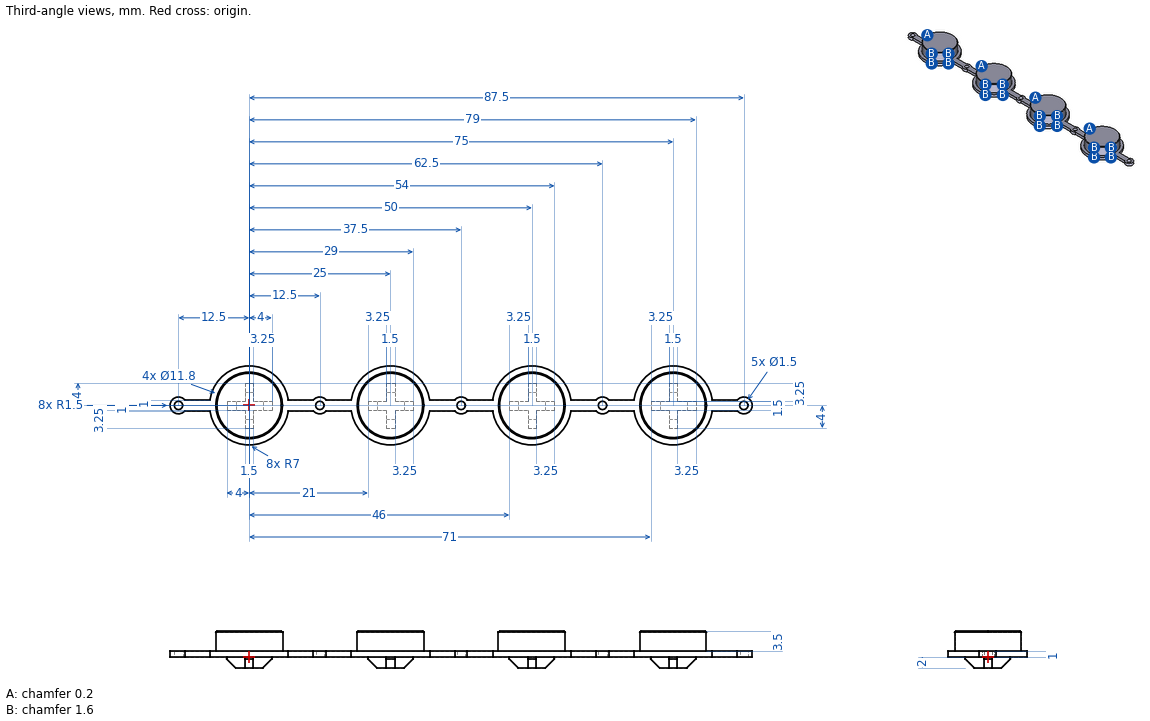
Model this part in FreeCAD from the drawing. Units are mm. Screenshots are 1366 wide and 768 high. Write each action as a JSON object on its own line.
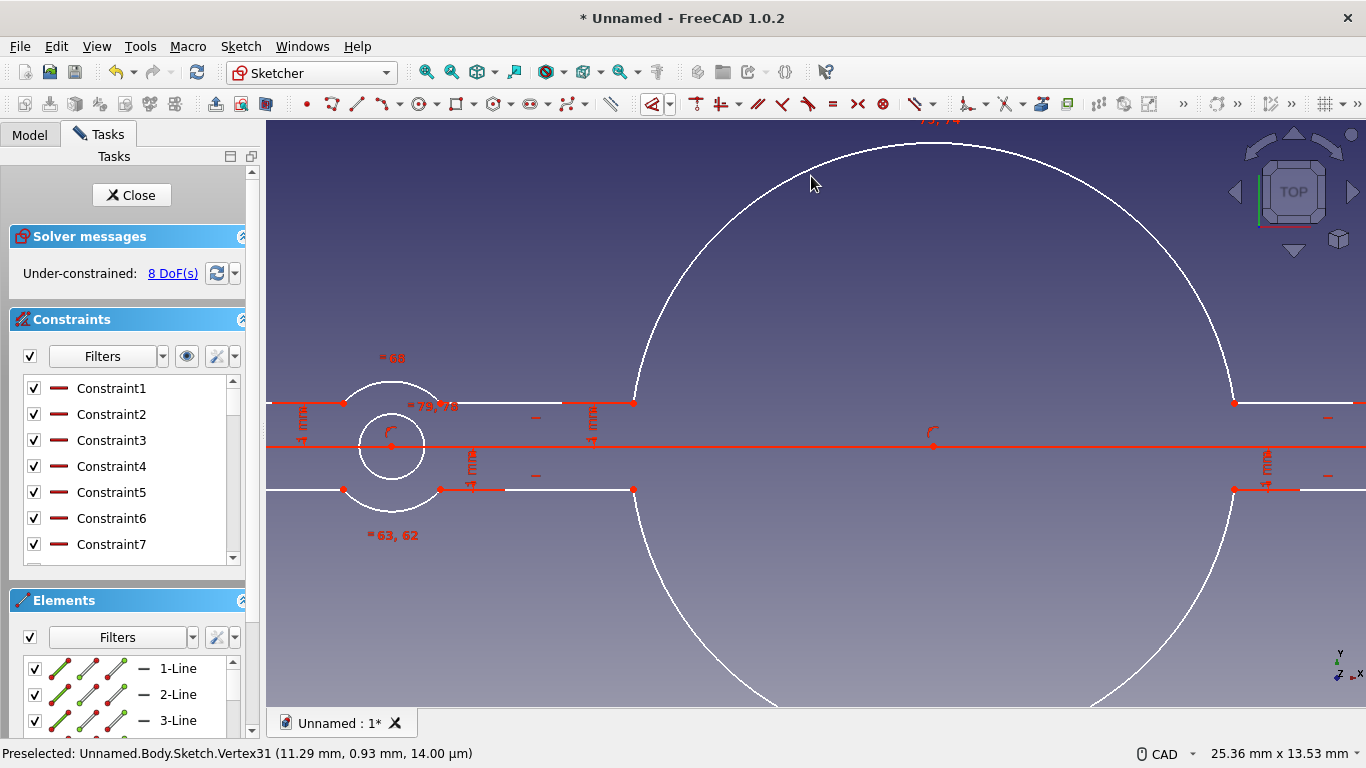
{"action": "scroll", "coordinate": [633, 408], "scroll_direction": "down", "scroll_amount": 10}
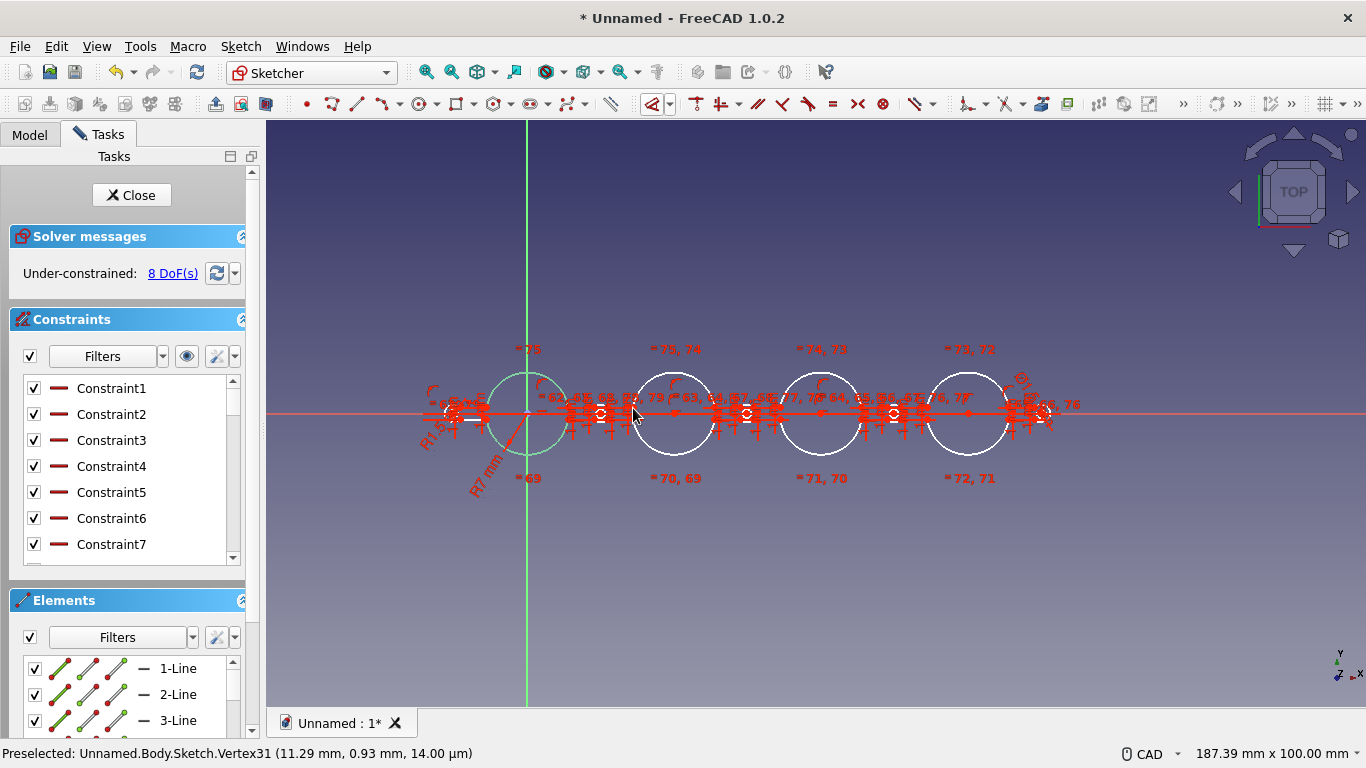
{"action": "left_click", "coordinate": [674, 414]}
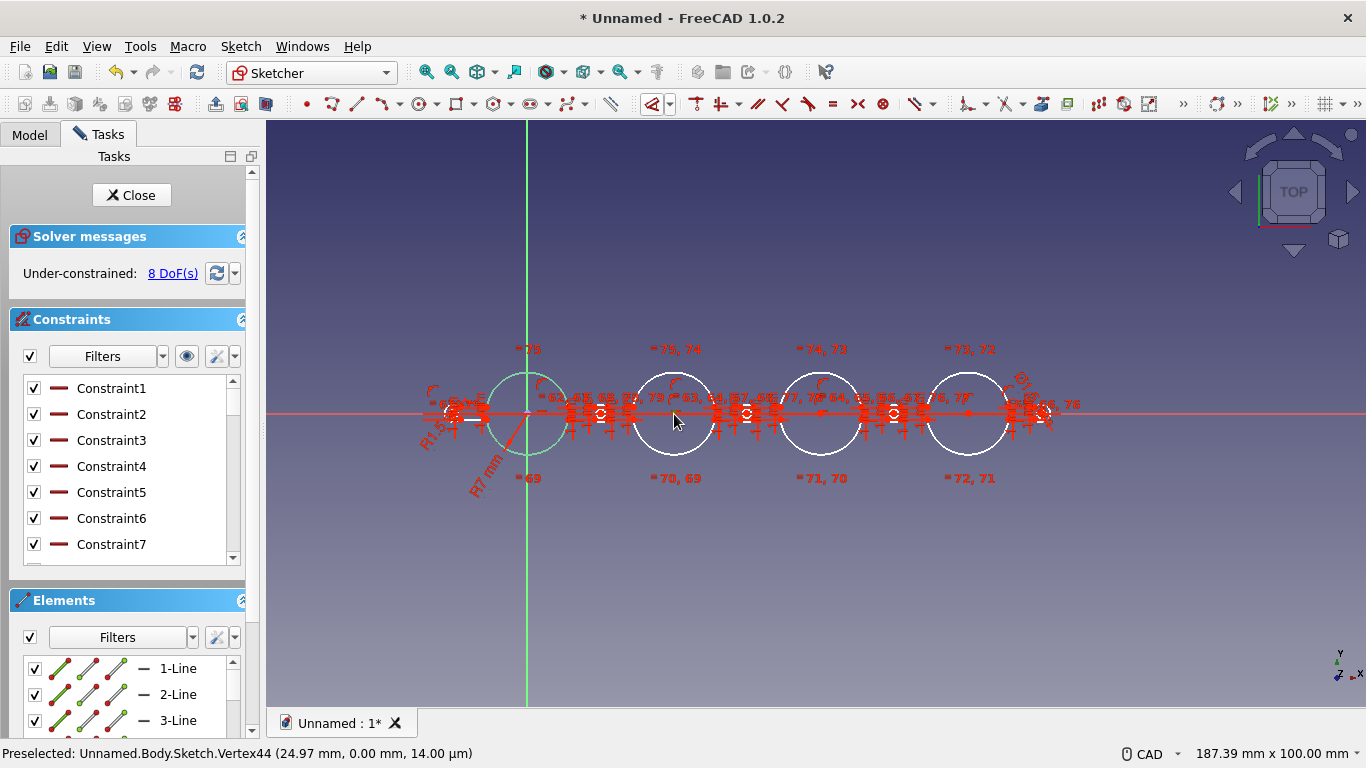
{"action": "key", "text": "l"}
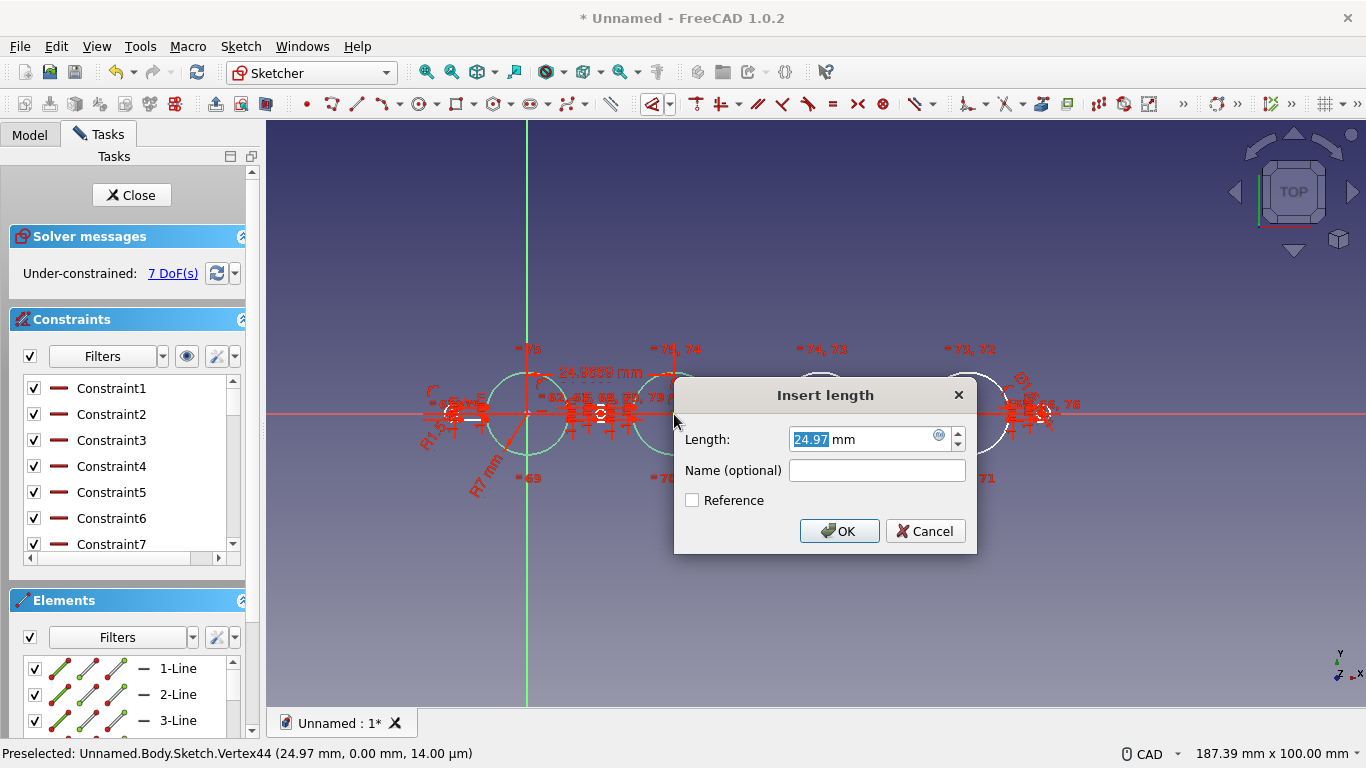
{"action": "type", "text": "25"}
{"action": "key", "text": "Return"}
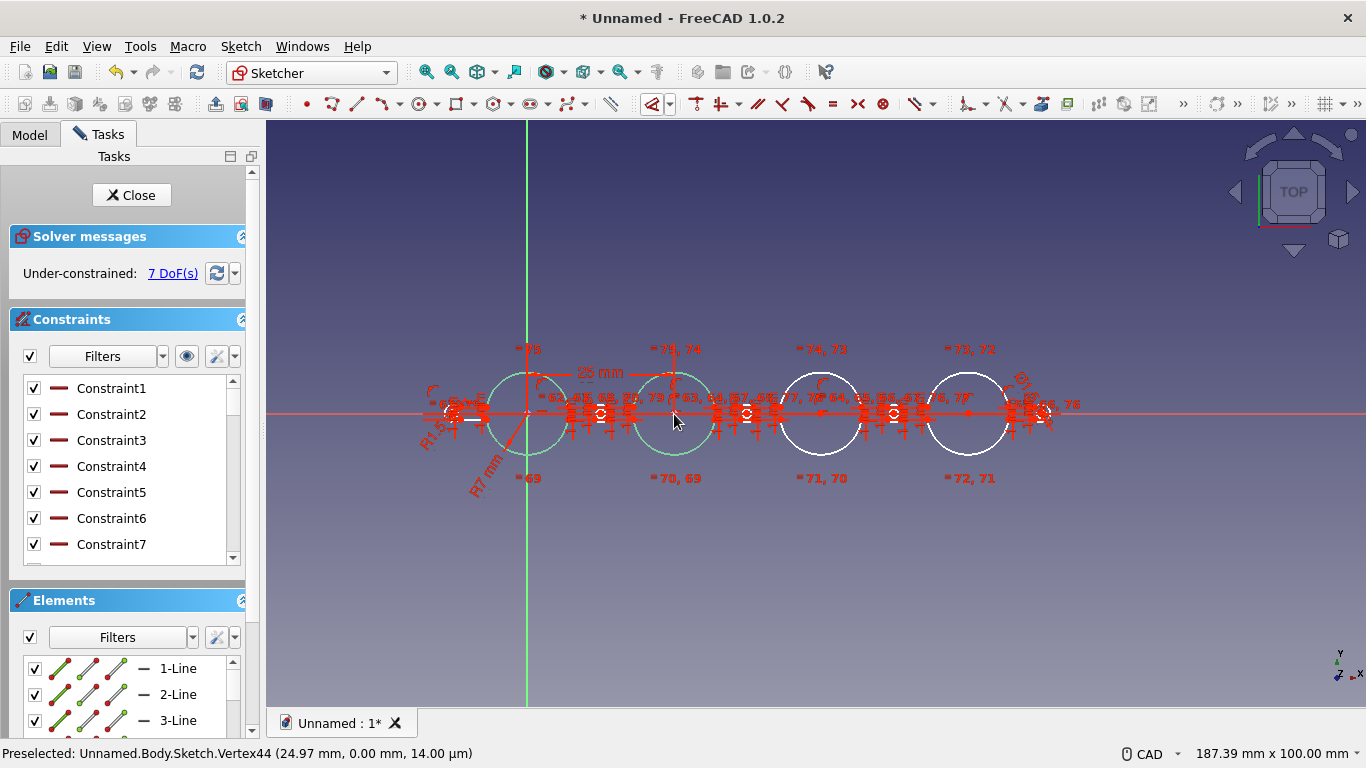
{"action": "left_click", "coordinate": [821, 414]}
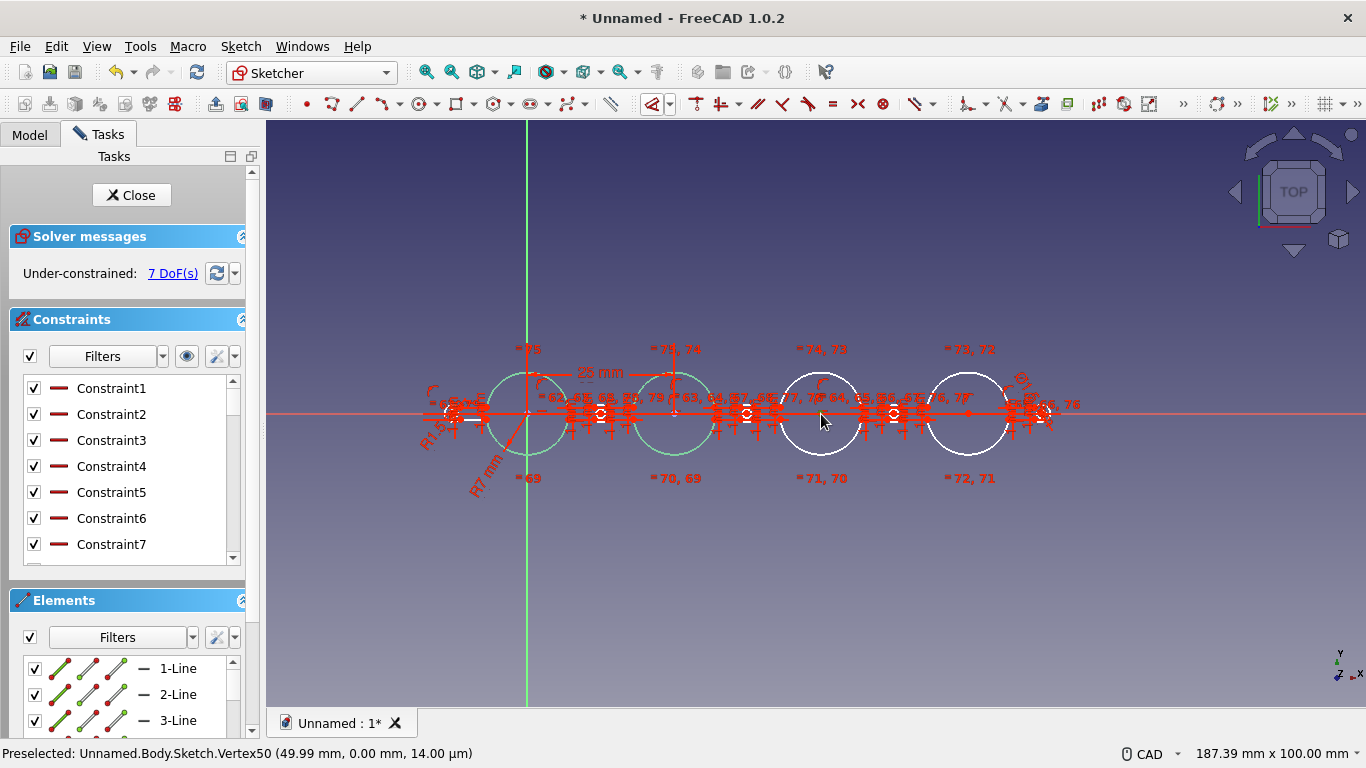
{"action": "key", "text": "l"}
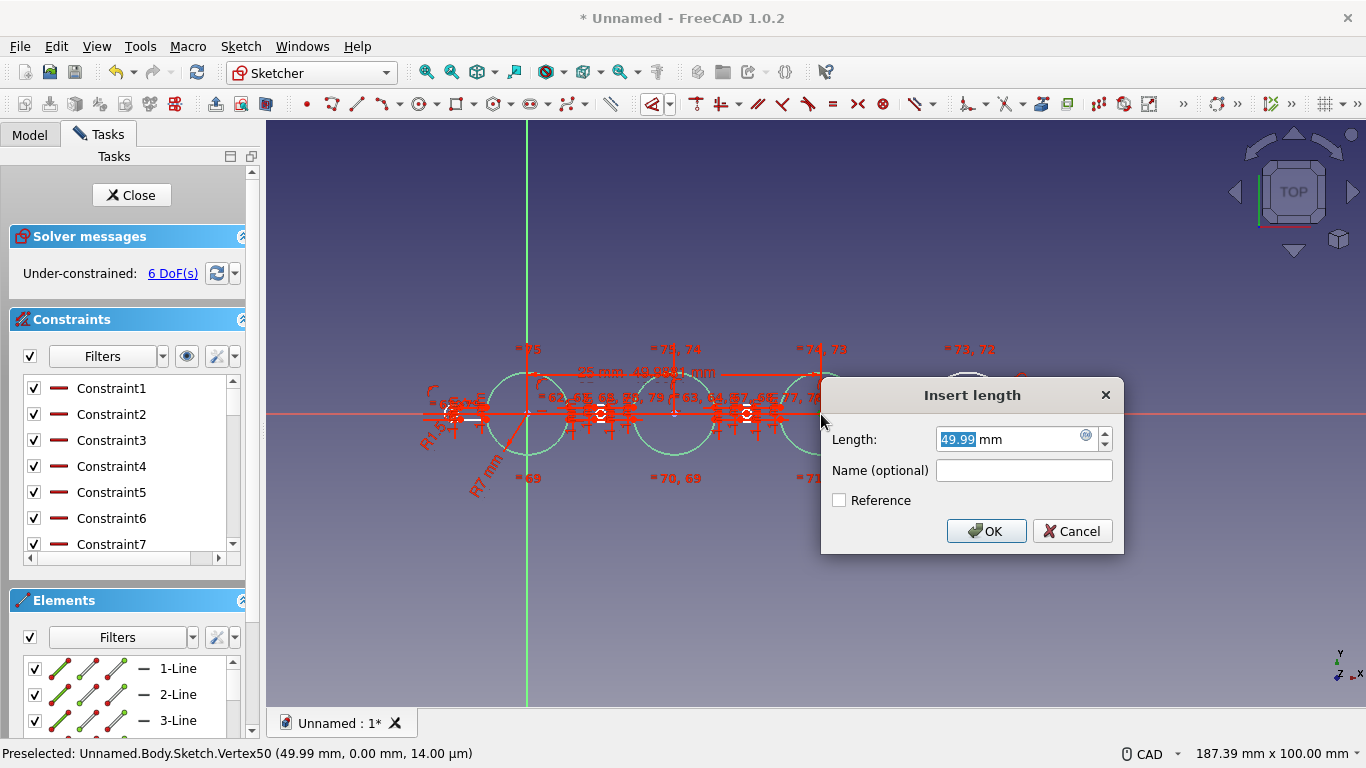
{"action": "type", "text": "50"}
{"action": "key", "text": "Return"}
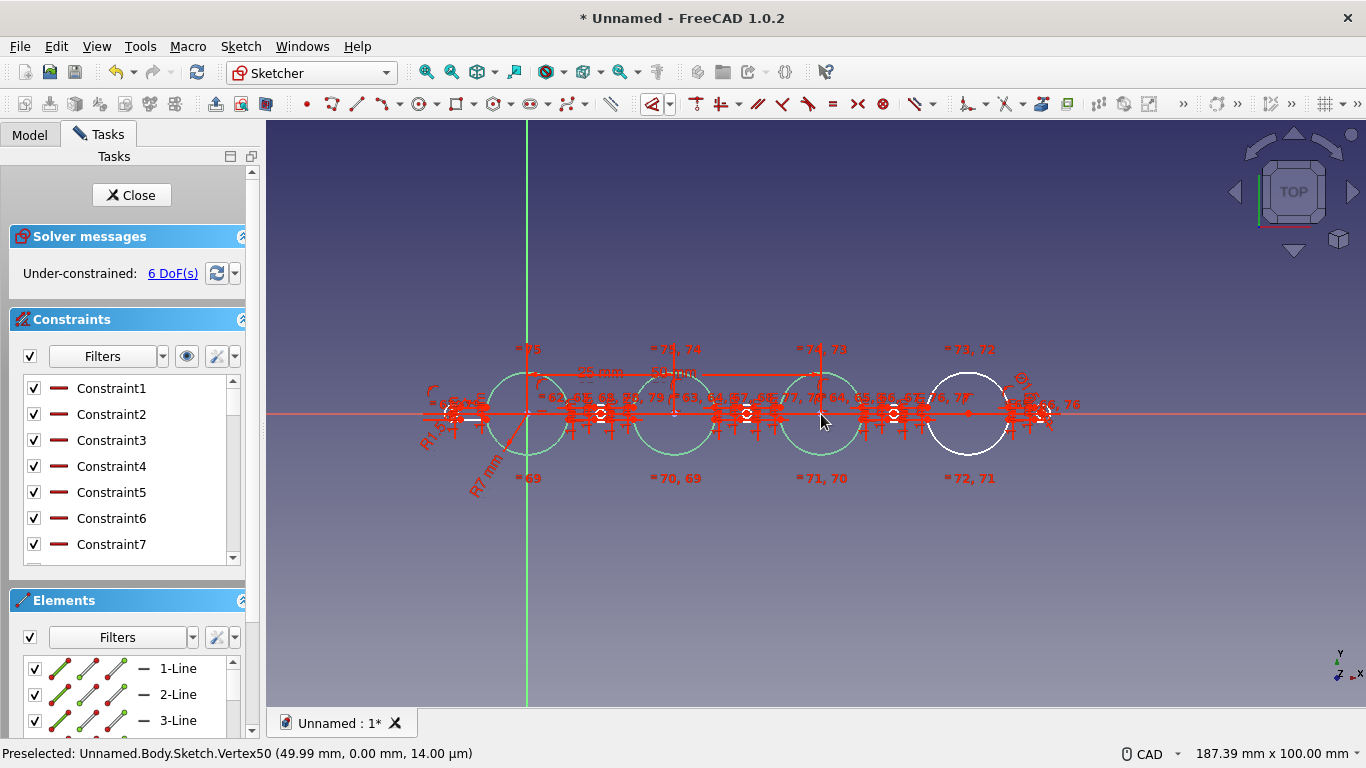
{"action": "left_click", "coordinate": [968, 414]}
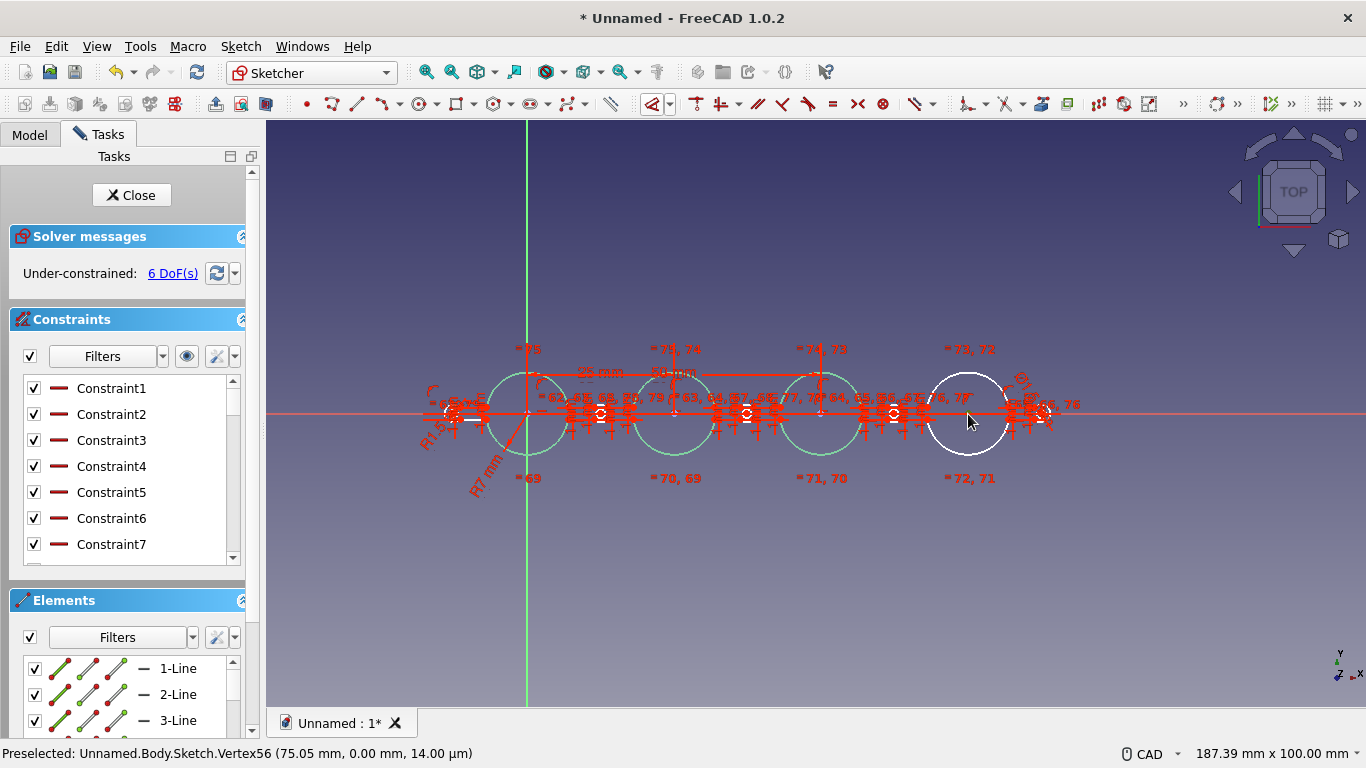
{"action": "key", "text": "l"}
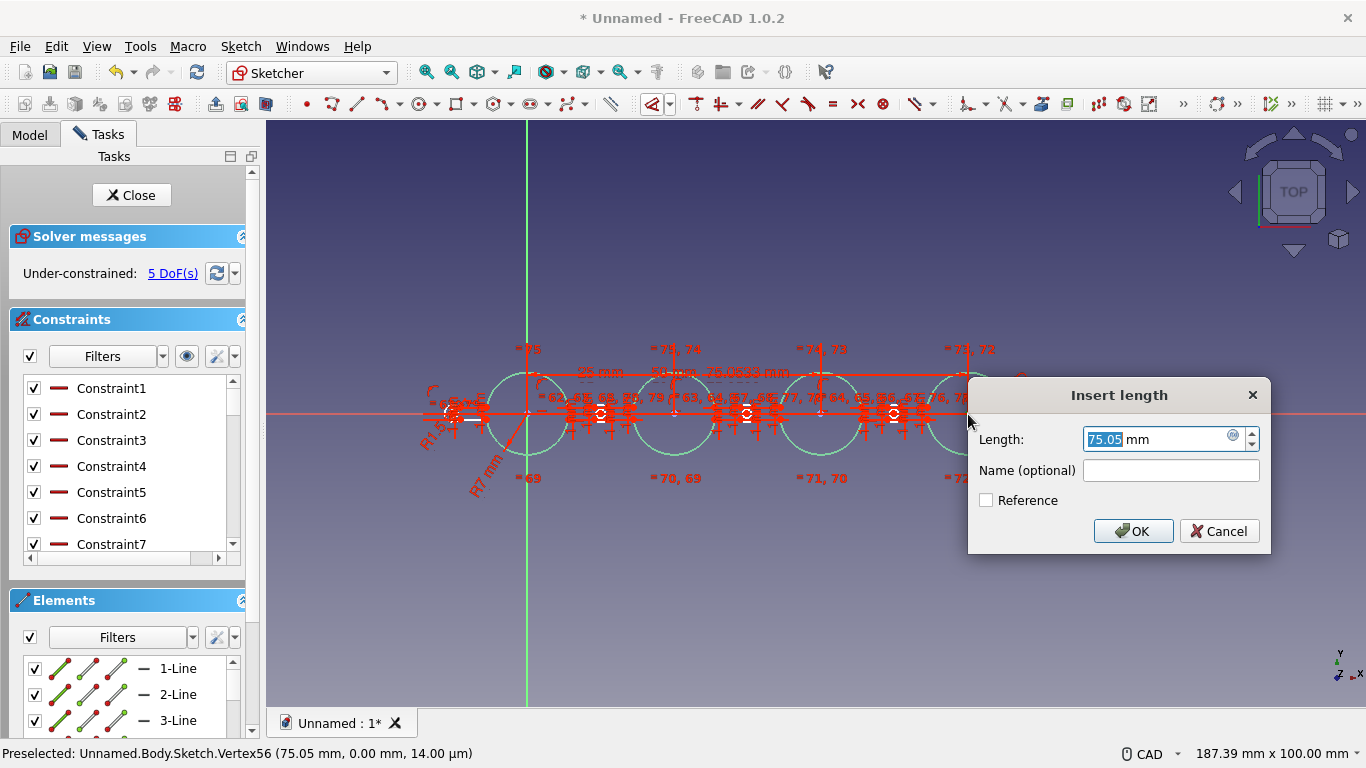
{"action": "type", "text": "75"}
{"action": "key", "text": "Return"}